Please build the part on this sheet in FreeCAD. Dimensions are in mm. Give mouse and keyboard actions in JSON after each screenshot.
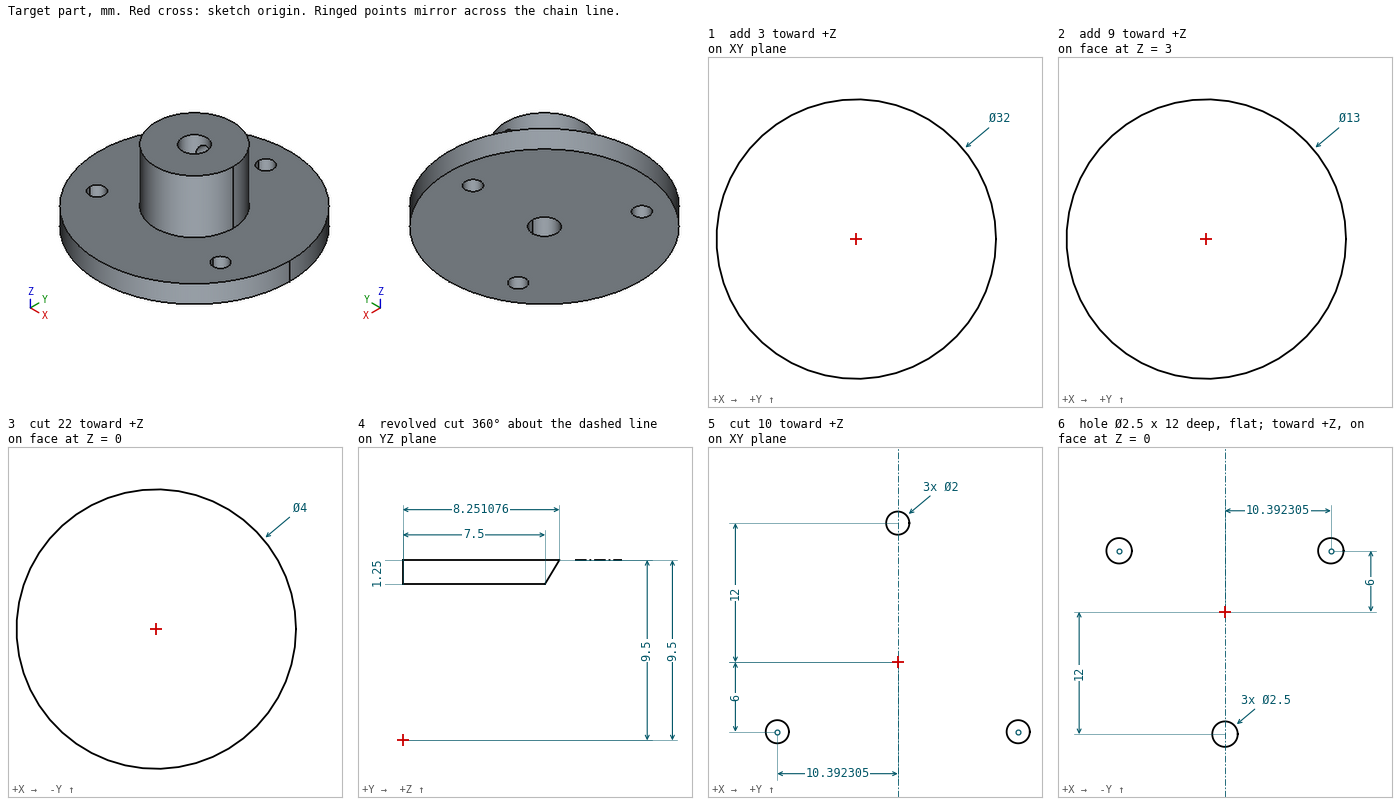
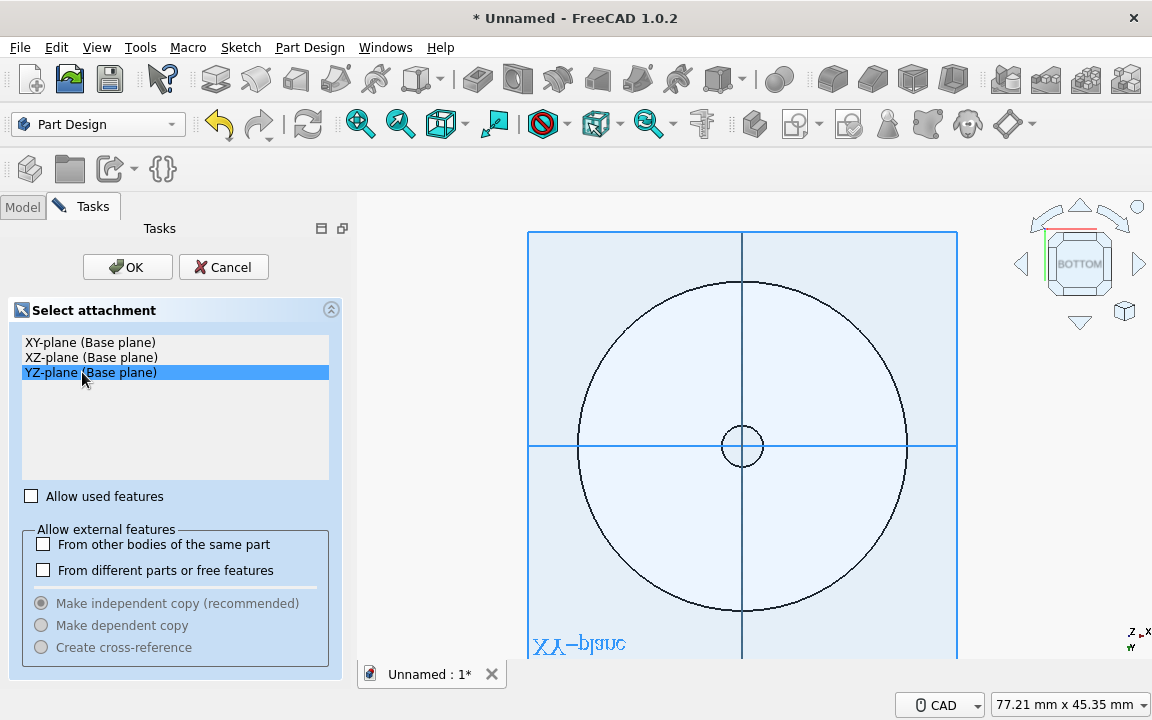
{"action": "left_click", "coordinate": [128, 267]}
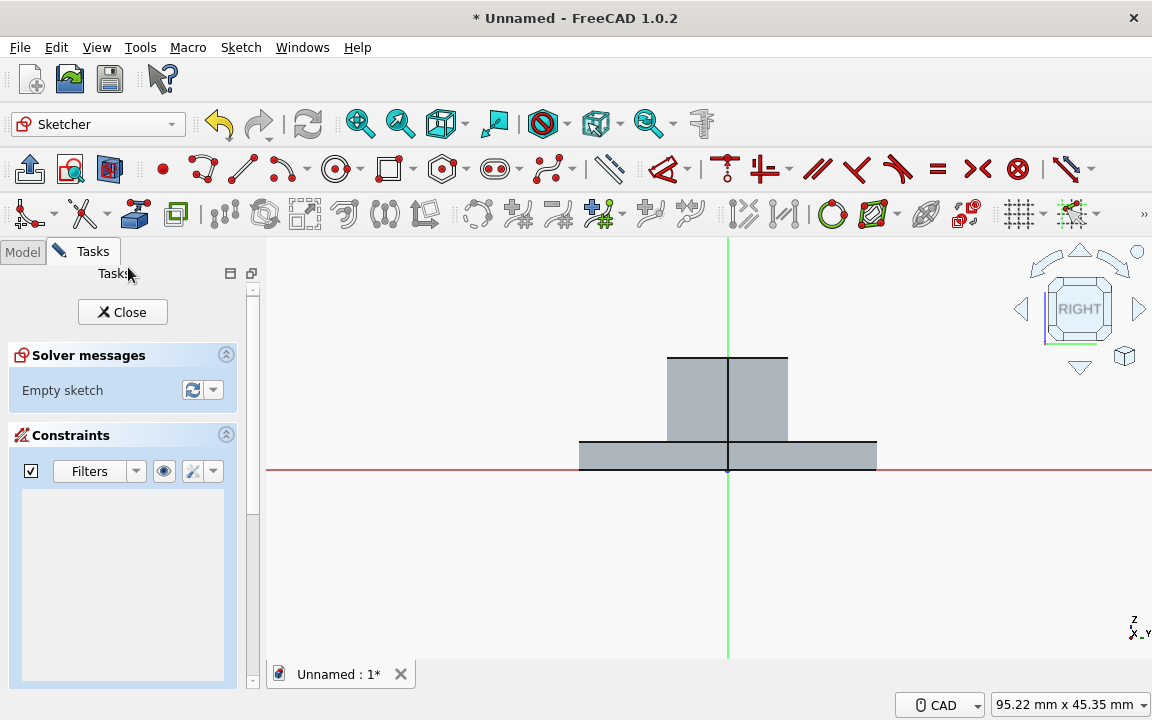
{"action": "left_click", "coordinate": [110, 170]}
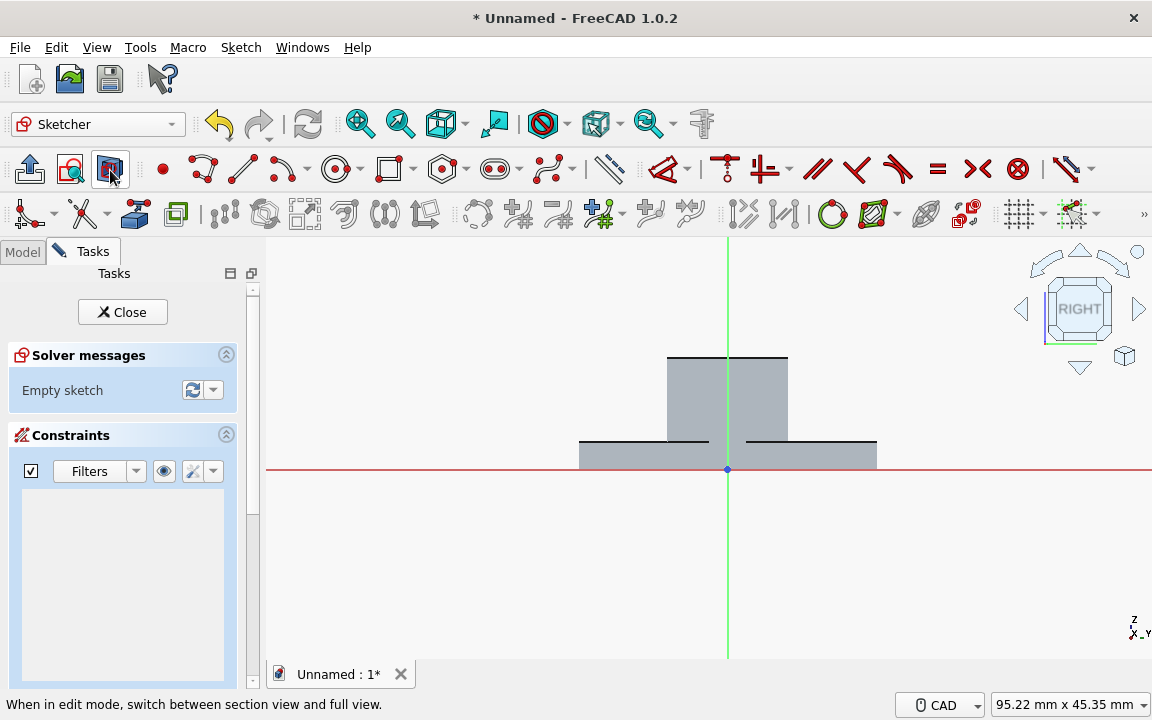
{"action": "scroll", "coordinate": [864, 412], "scroll_direction": "up", "scroll_amount": 5}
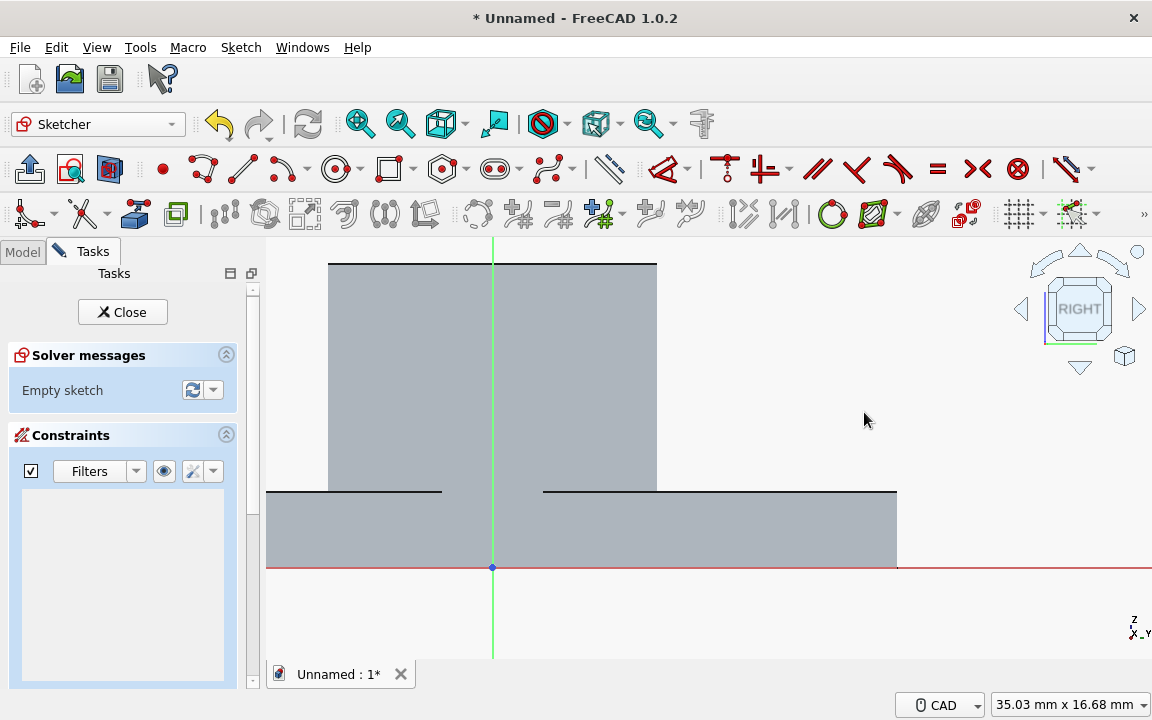
{"action": "left_click", "coordinate": [204, 170]}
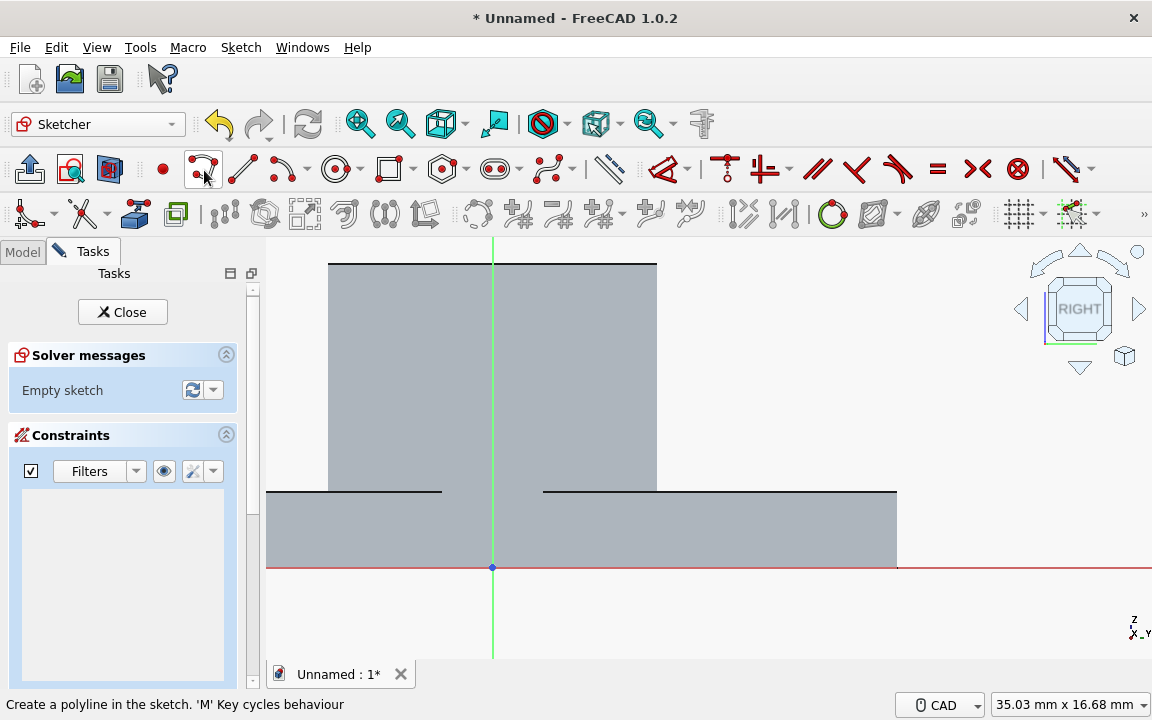
{"action": "left_click", "coordinate": [493, 359]}
{"action": "left_click", "coordinate": [682, 359]}
{"action": "left_click", "coordinate": [701, 327]}
{"action": "left_click", "coordinate": [502, 327]}
{"action": "left_click", "coordinate": [493, 360]}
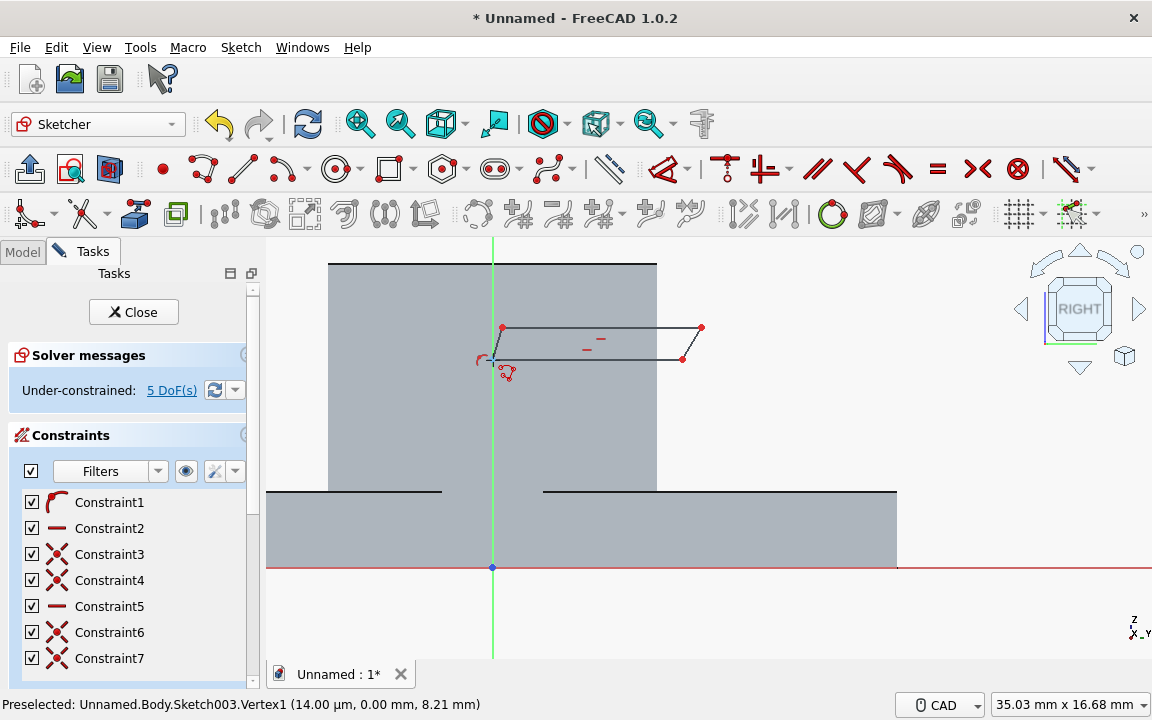
{"action": "left_click", "coordinate": [244, 170]}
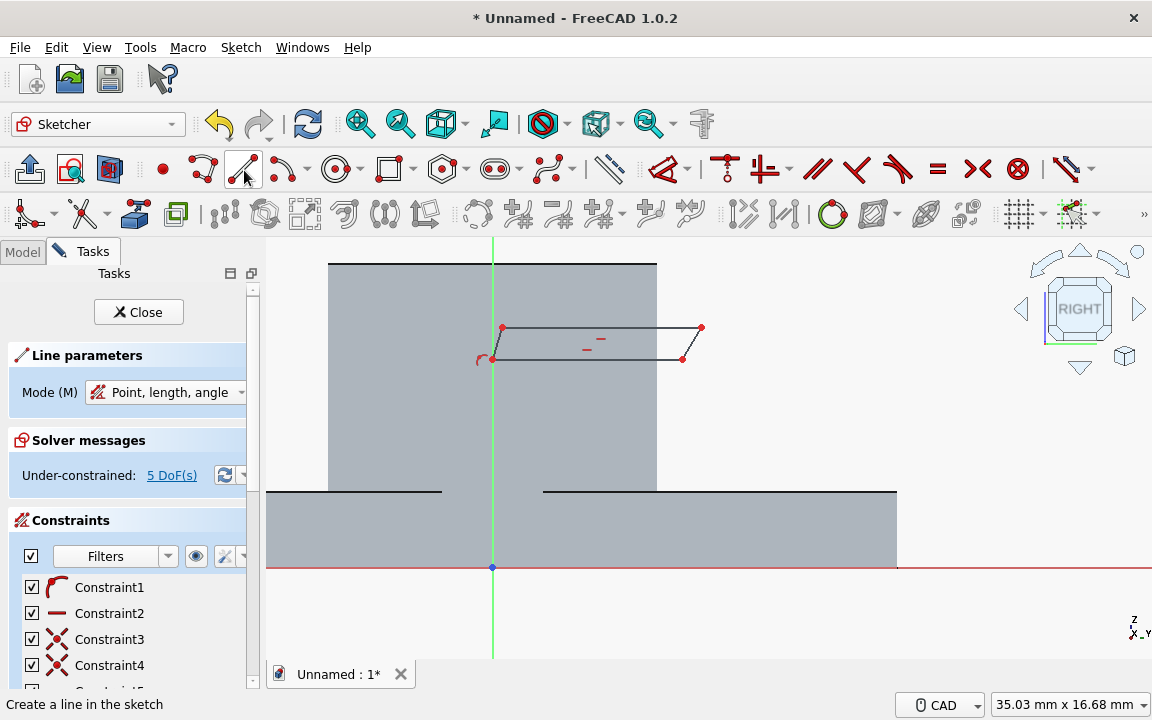
{"action": "left_click", "coordinate": [722, 327]}
{"action": "left_click", "coordinate": [785, 327]}
{"action": "key", "text": "Escape"}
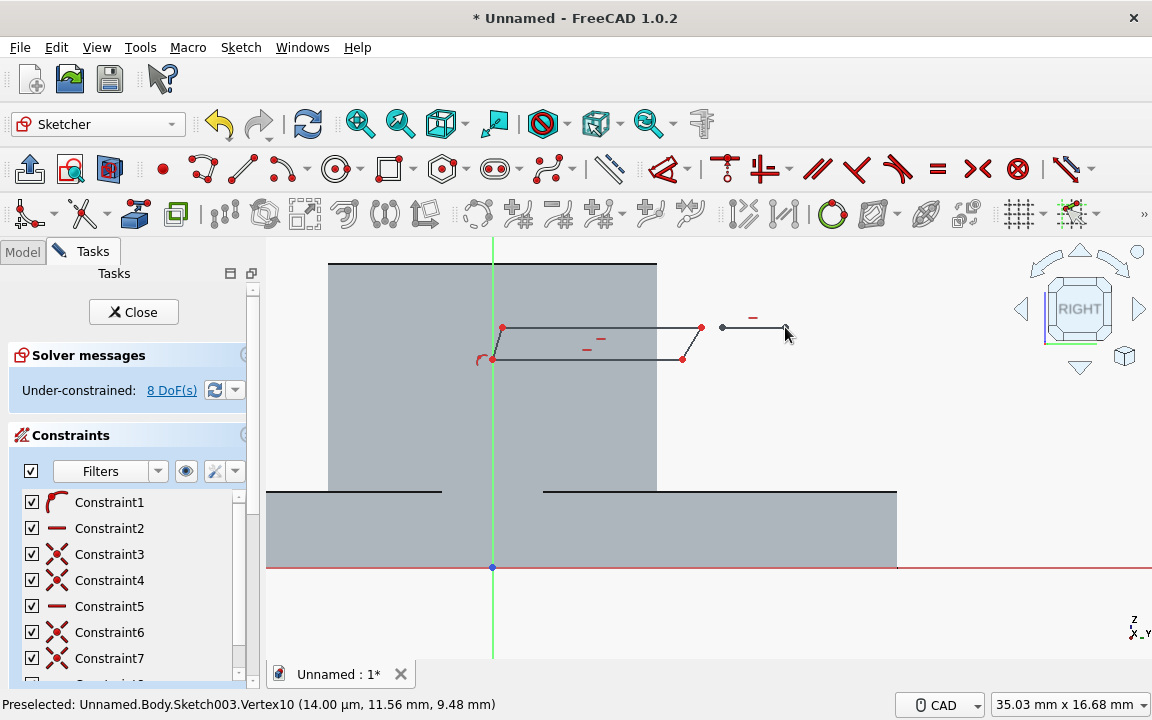
{"action": "left_click", "coordinate": [741, 328]}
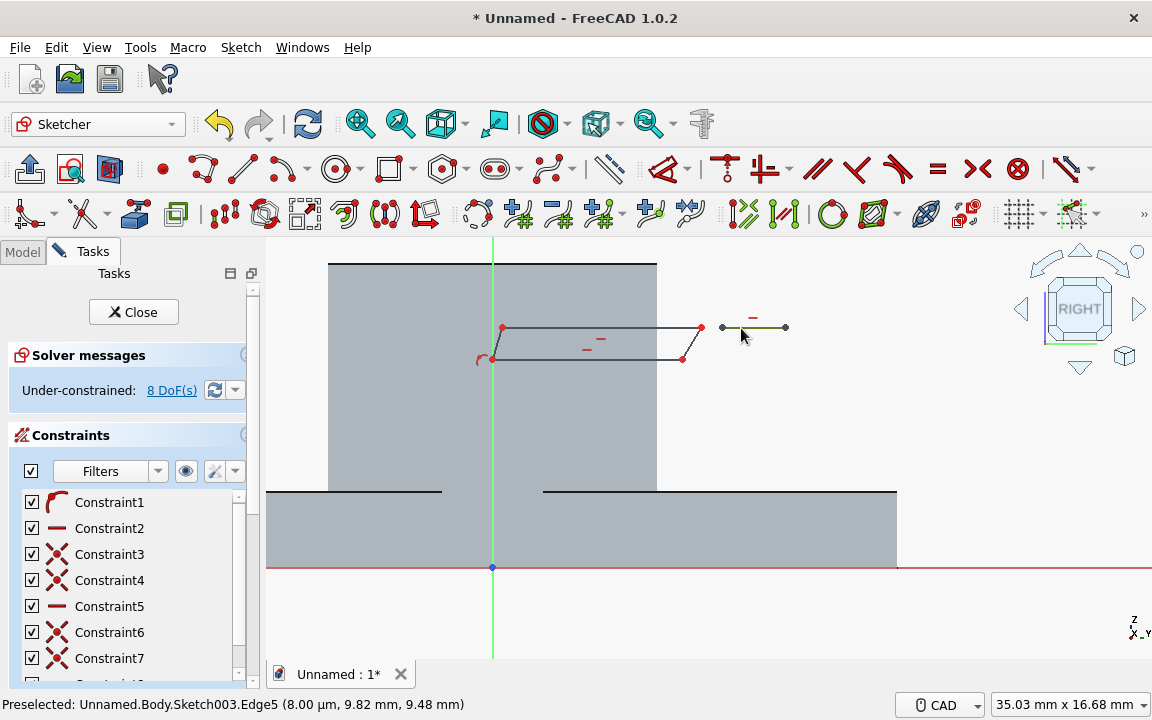
{"action": "left_click", "coordinate": [610, 170]}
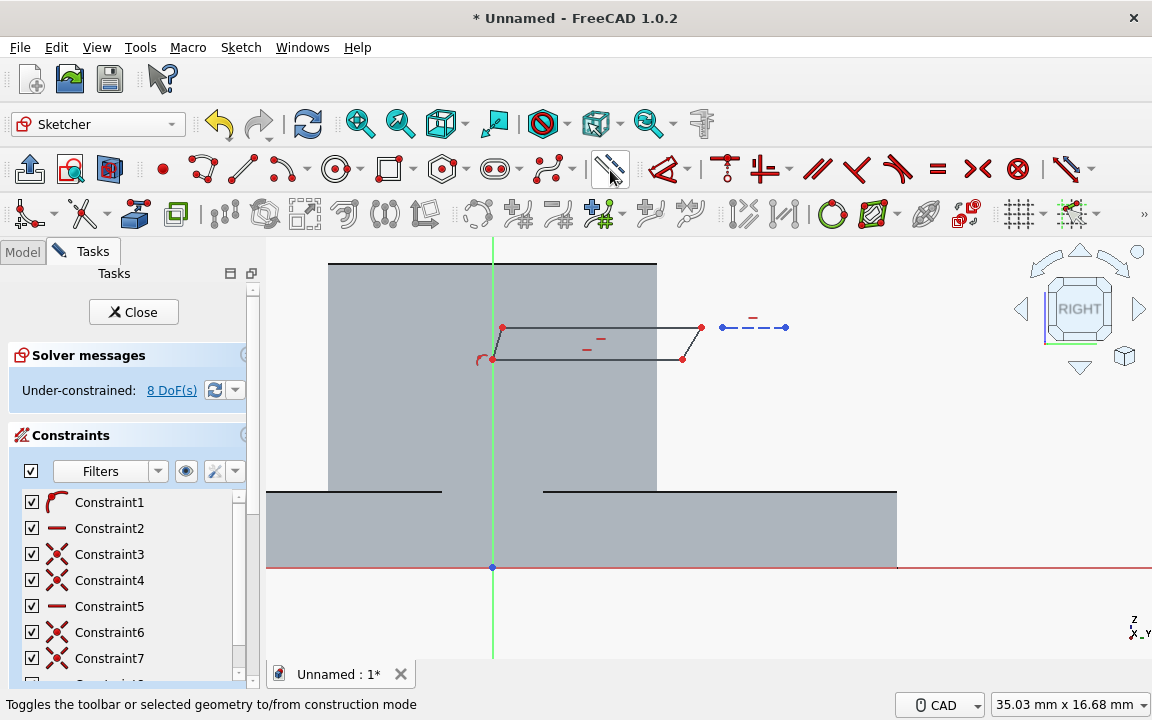
{"action": "scroll", "coordinate": [495, 350], "scroll_direction": "up", "scroll_amount": 2}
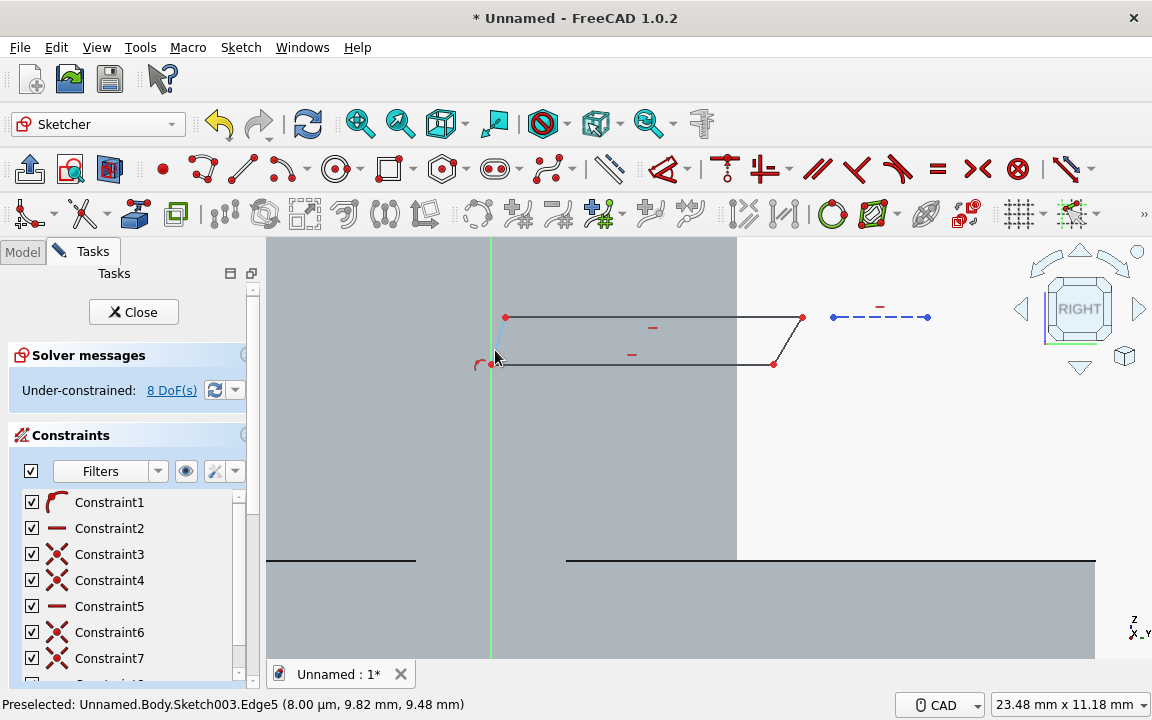
{"action": "left_click", "coordinate": [496, 350]}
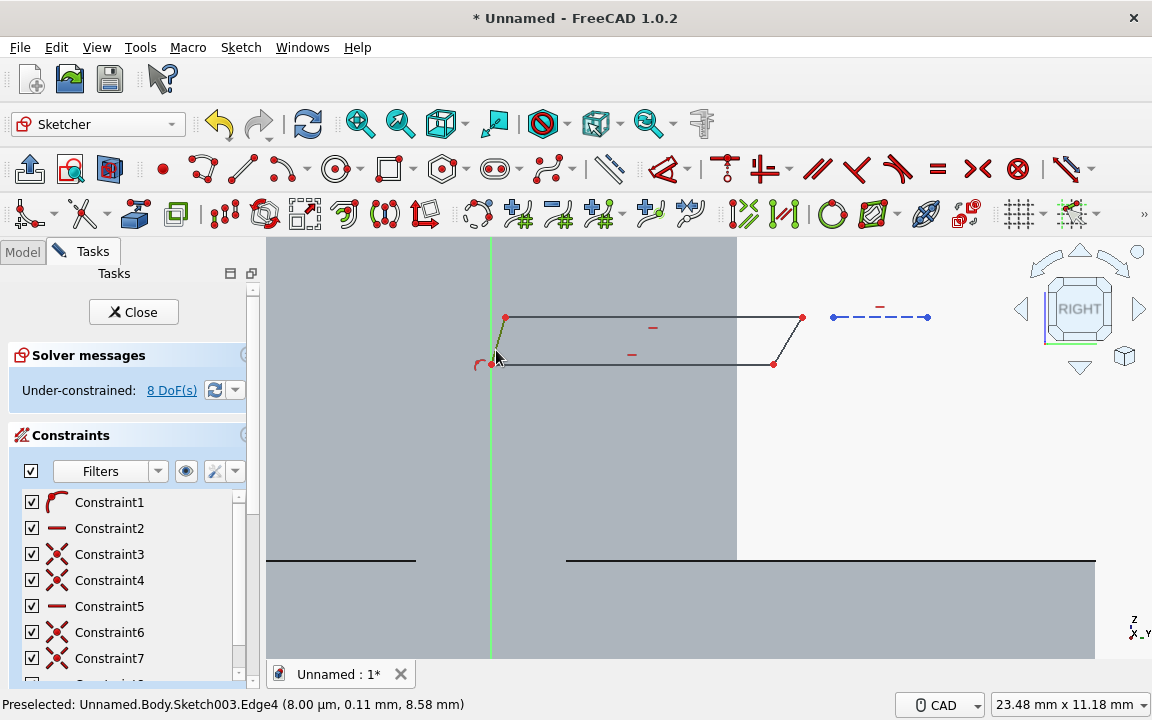
{"action": "left_click", "coordinate": [792, 170]}